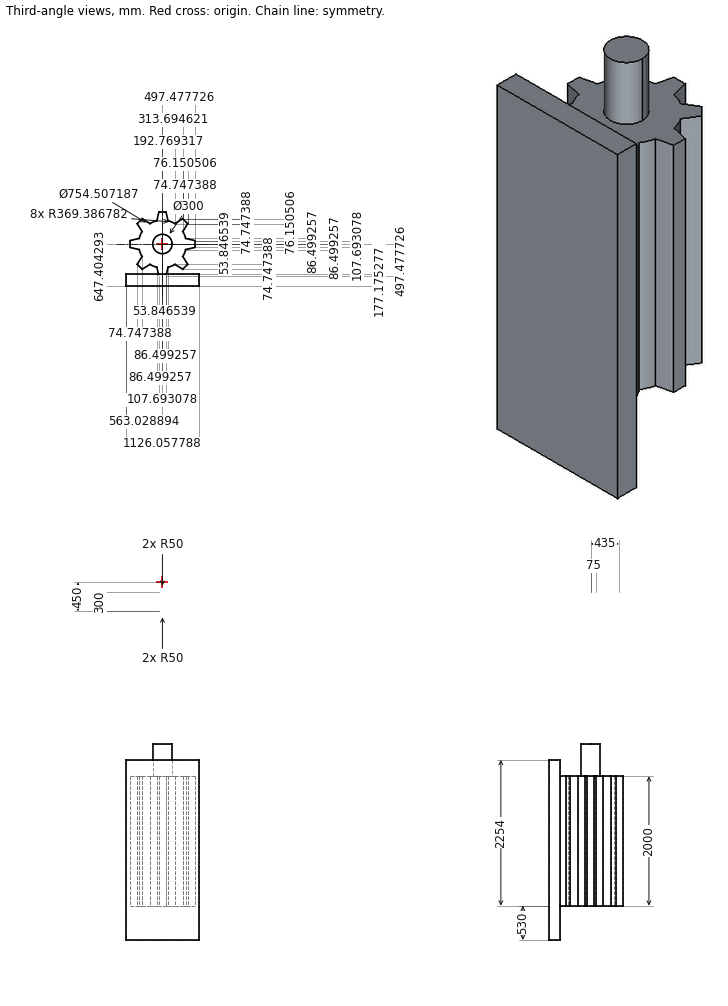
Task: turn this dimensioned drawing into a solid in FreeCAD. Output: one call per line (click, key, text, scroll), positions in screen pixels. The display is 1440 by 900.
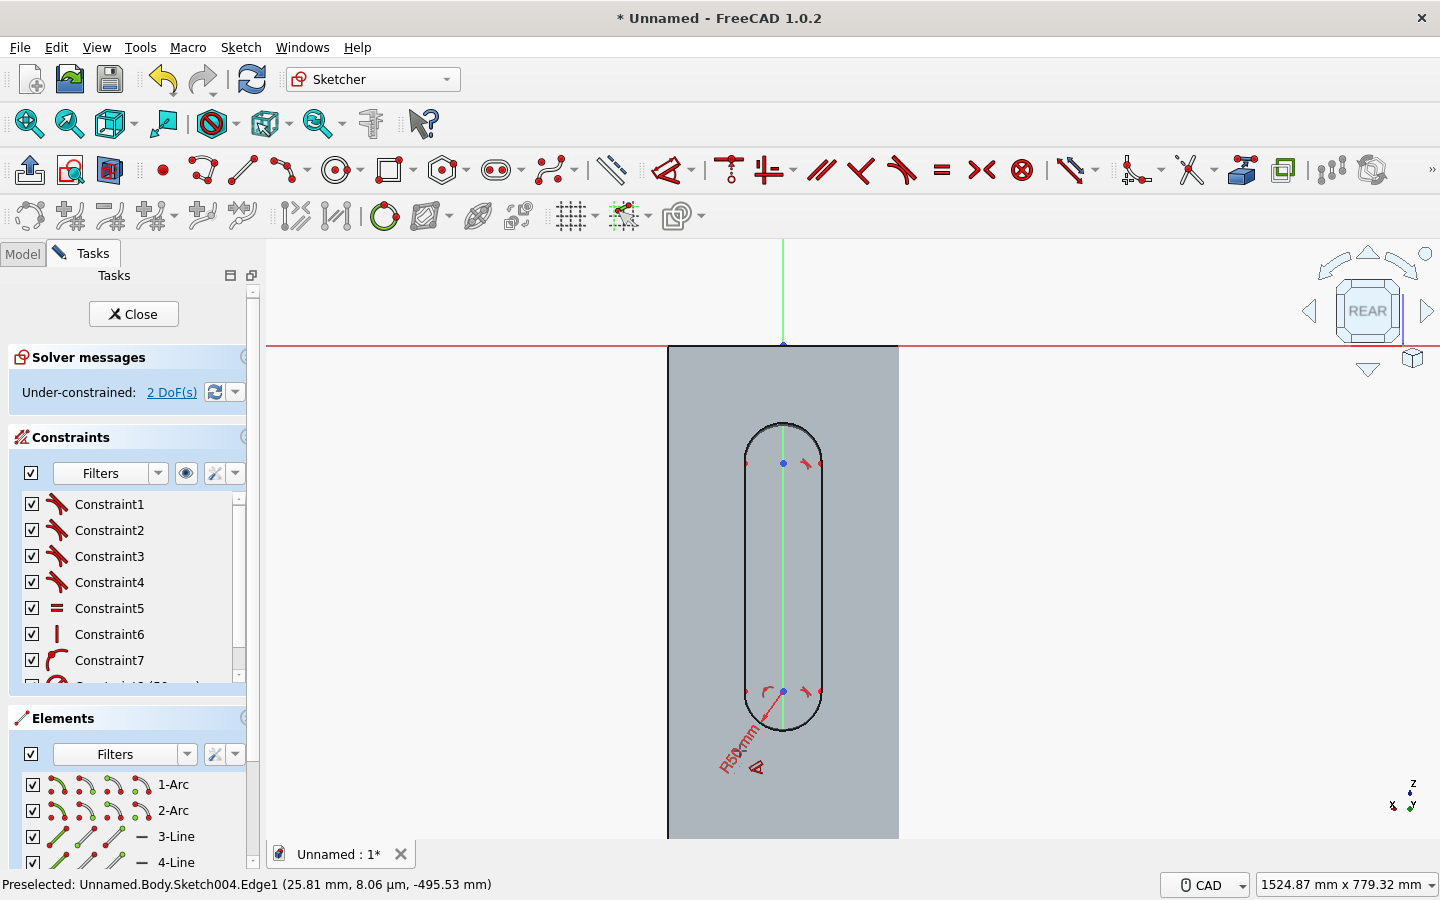
click(745, 623)
click(711, 578)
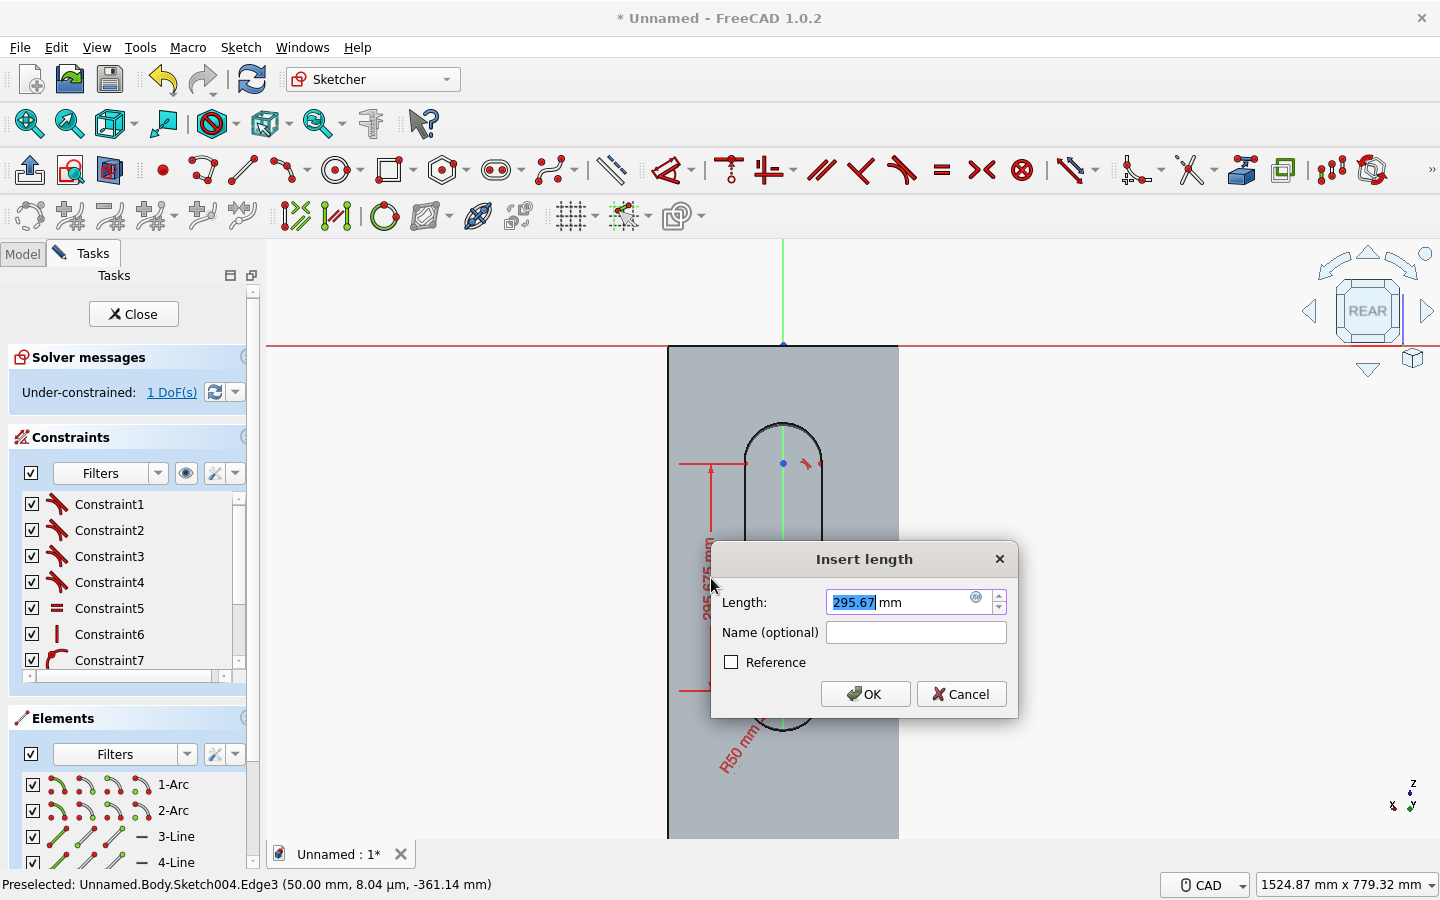
text(300)
key(Return)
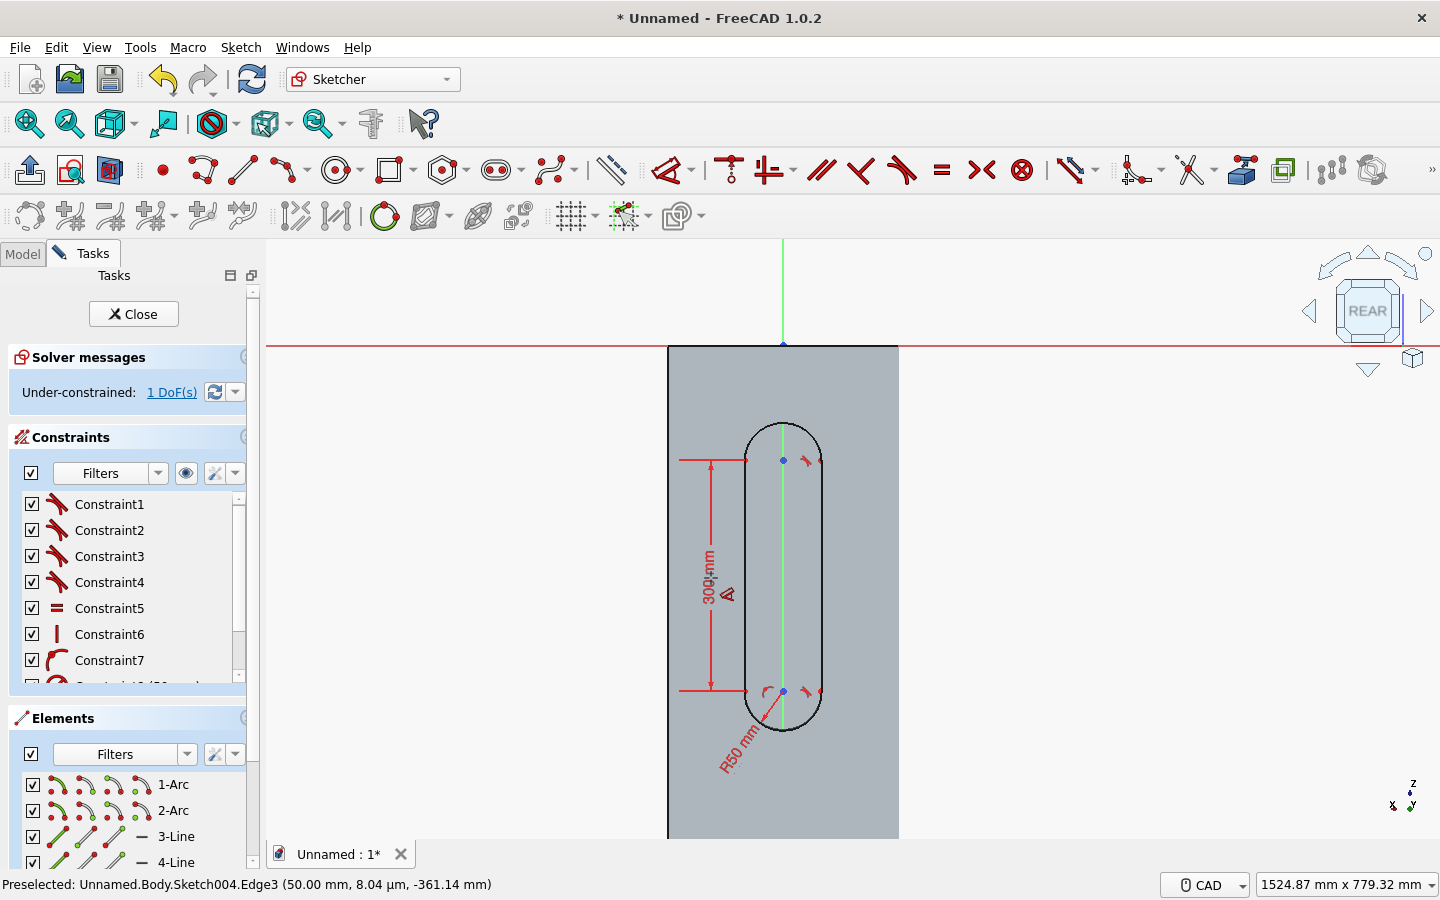
click(745, 691)
click(711, 519)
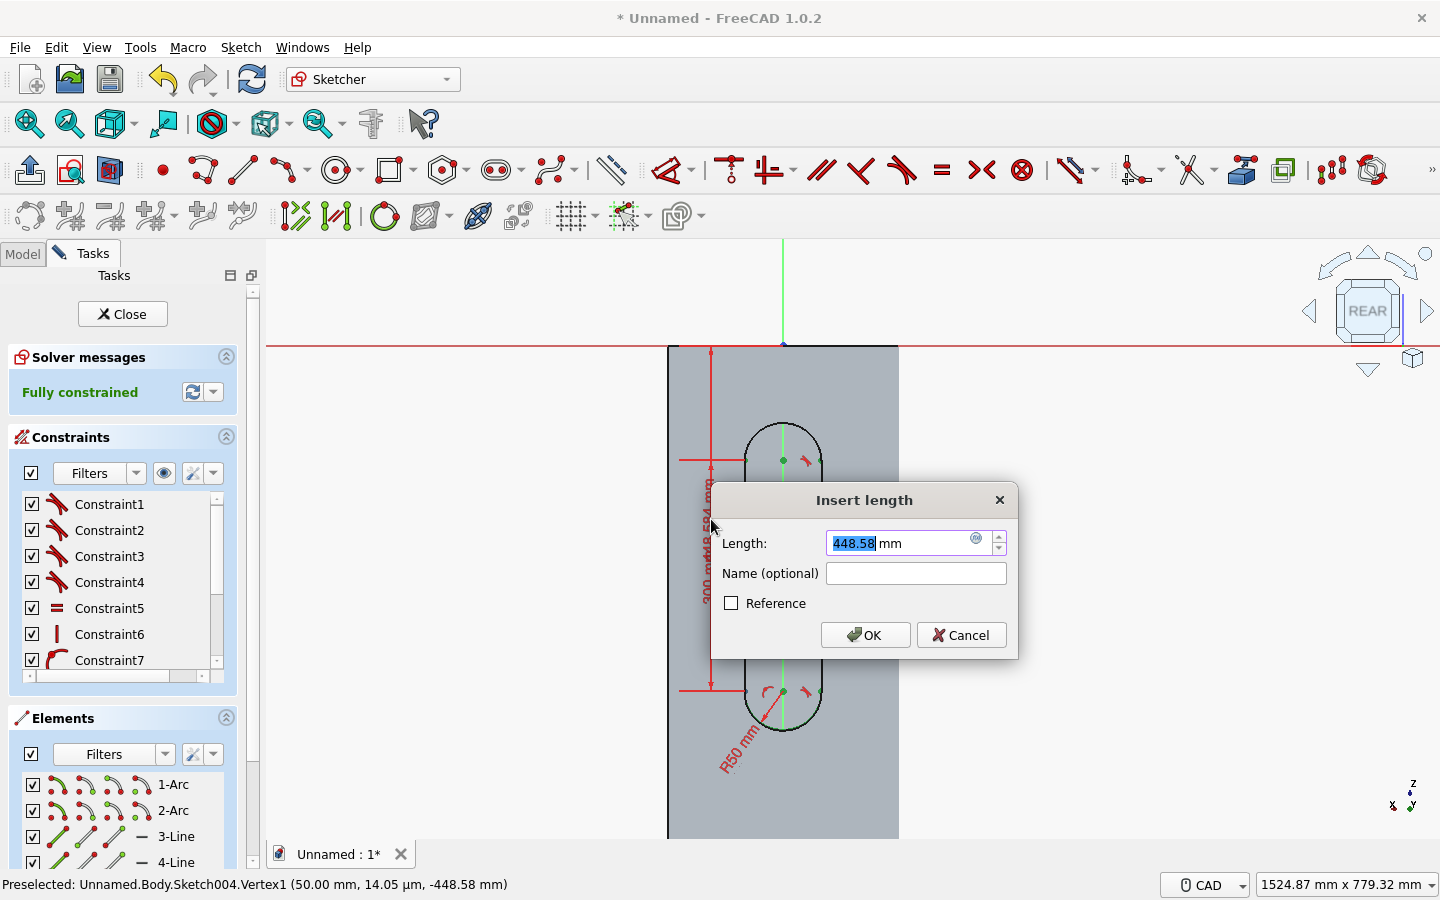
text(450)
key(Return)
key(Escape)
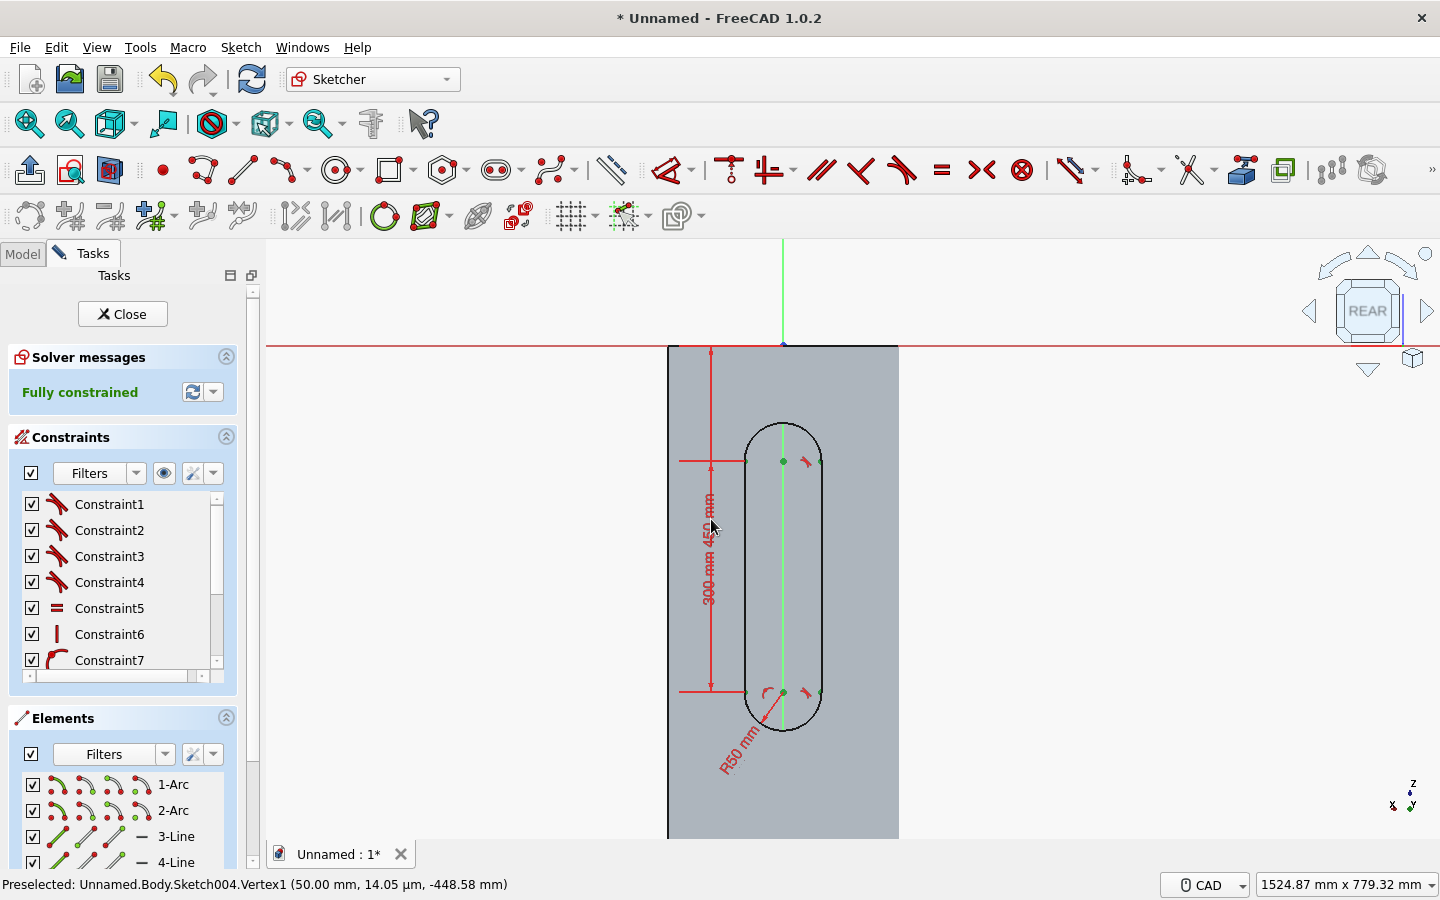
click(123, 314)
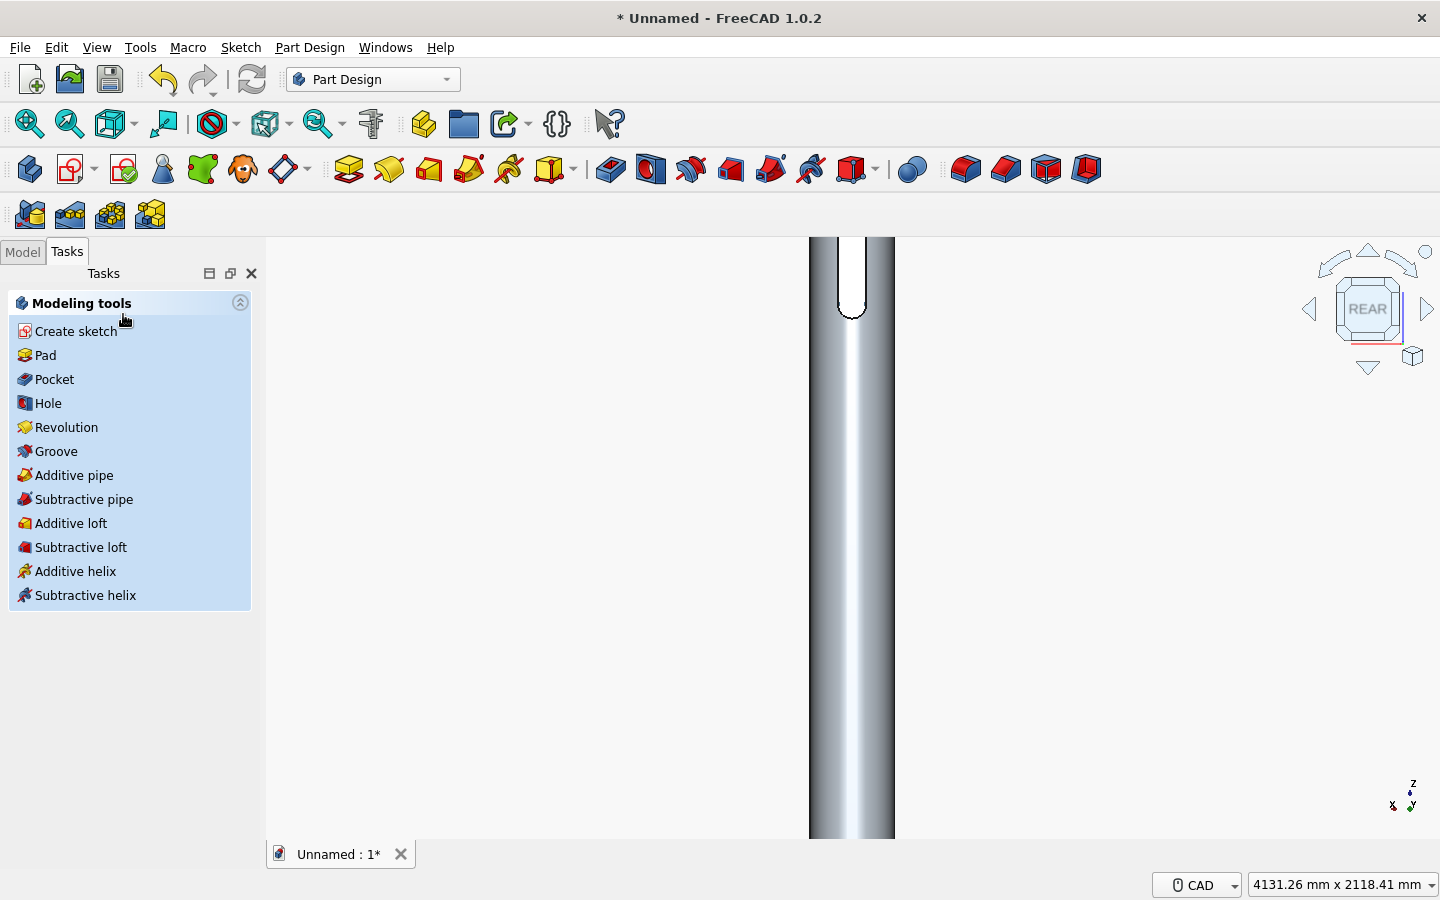
click(350, 170)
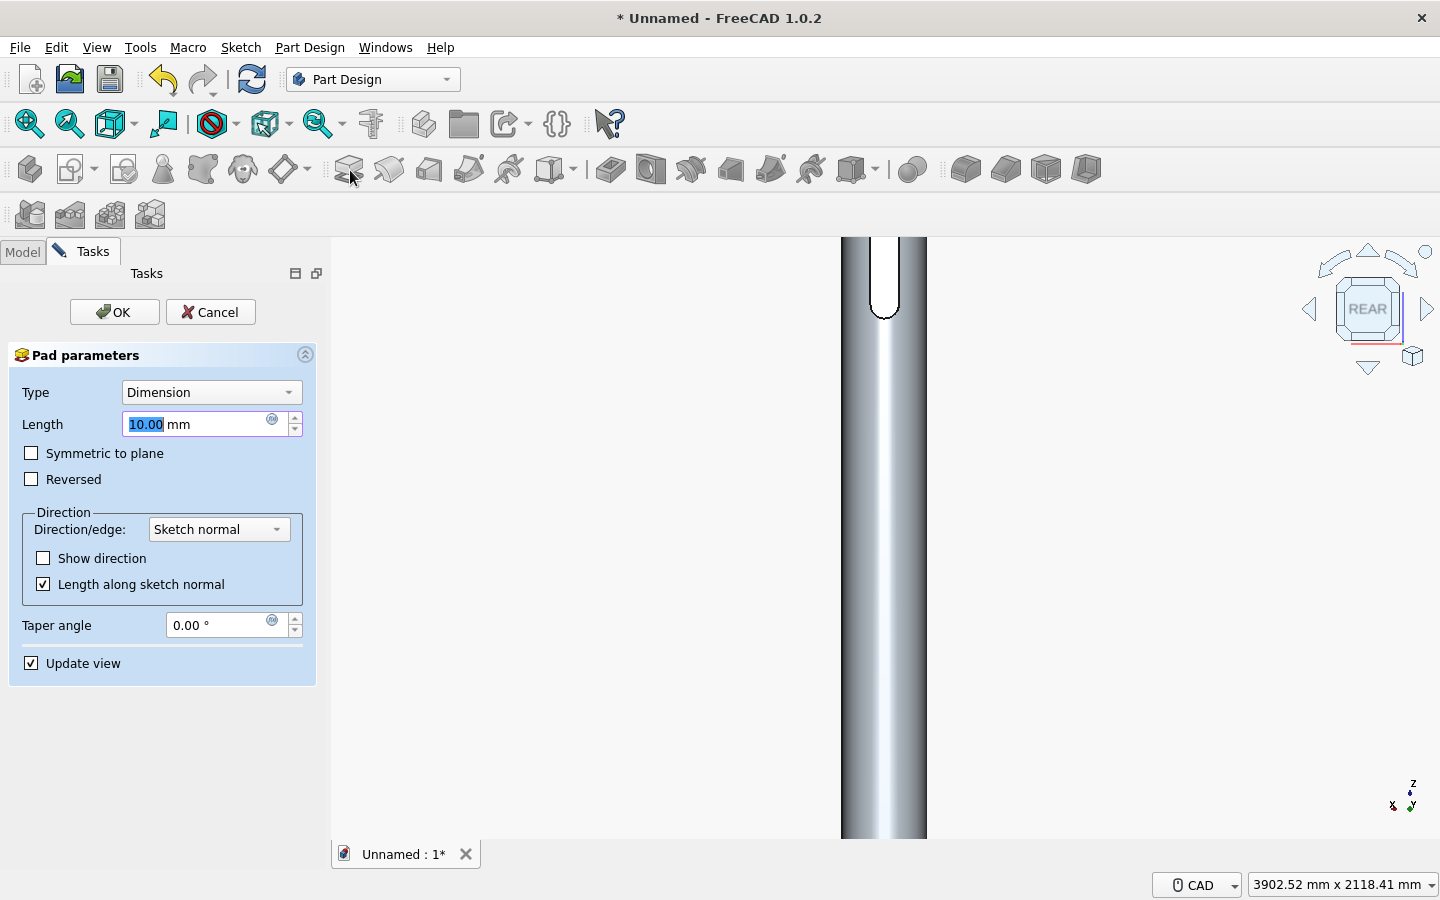
text(75)
key(Tab)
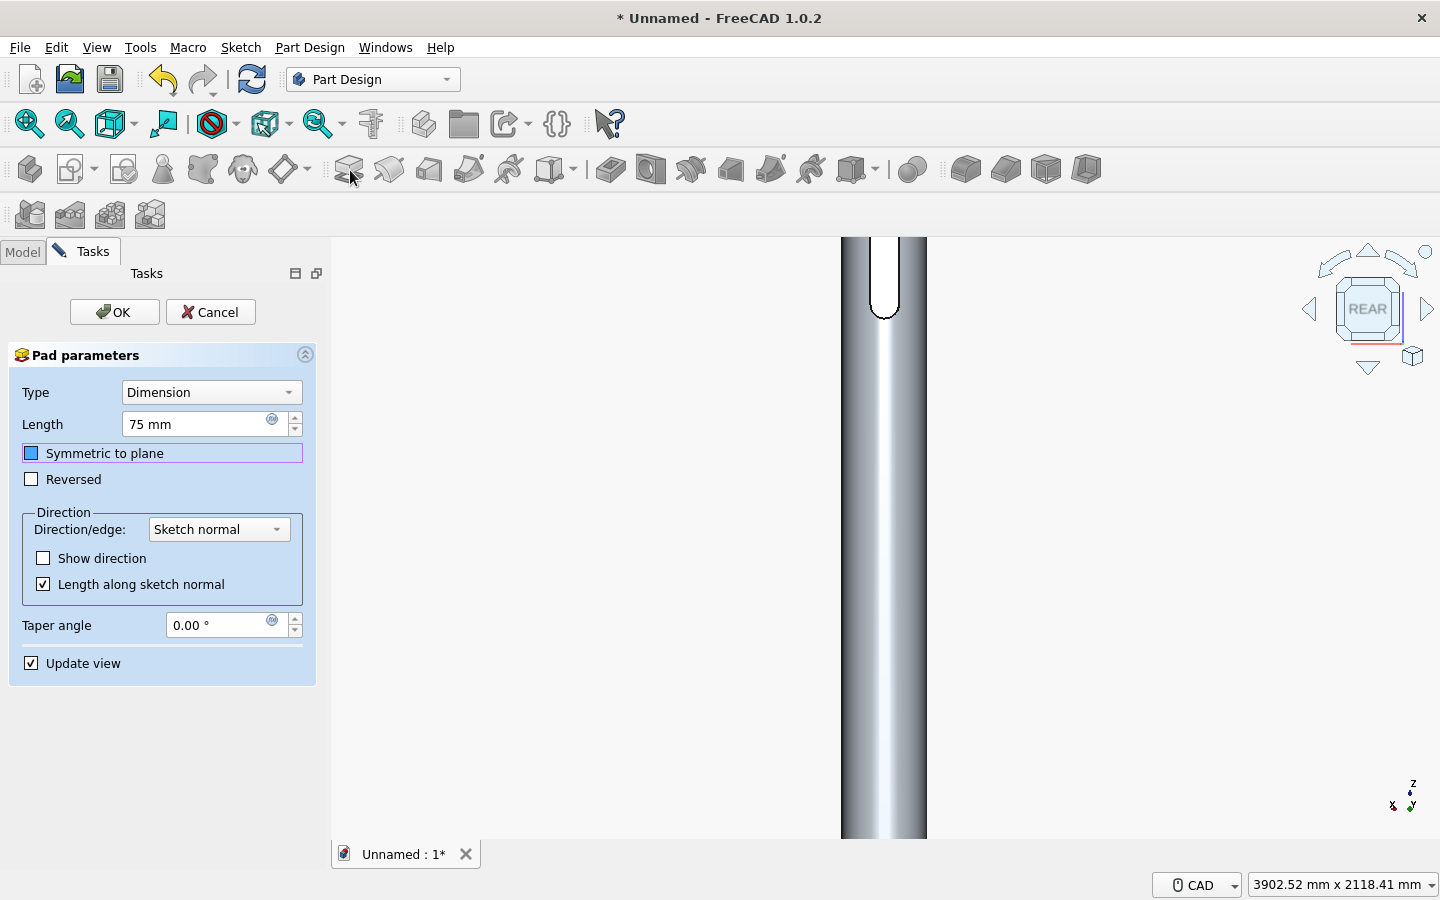
click(115, 312)